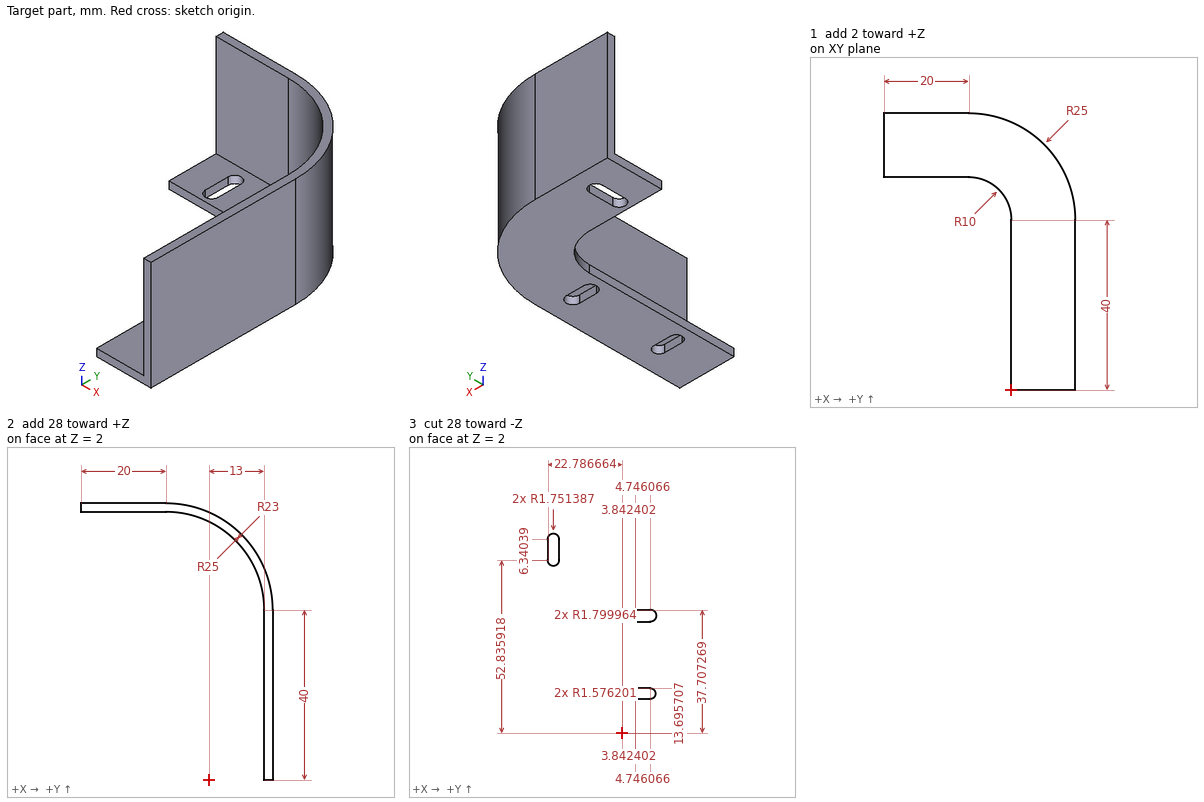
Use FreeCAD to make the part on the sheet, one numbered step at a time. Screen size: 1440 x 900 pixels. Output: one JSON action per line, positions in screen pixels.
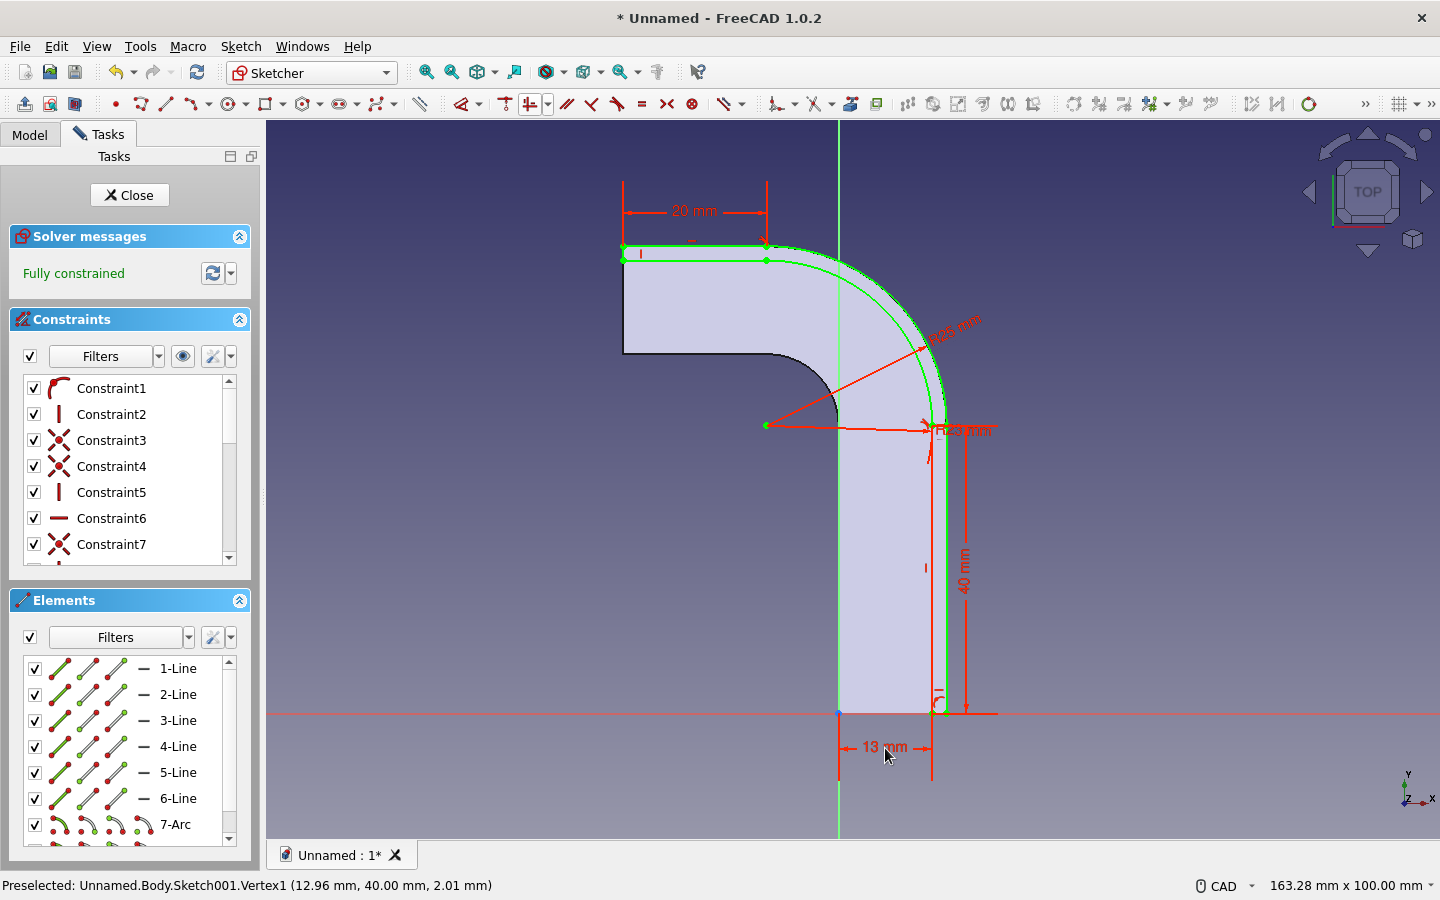
{"action": "left_click", "coordinate": [130, 195]}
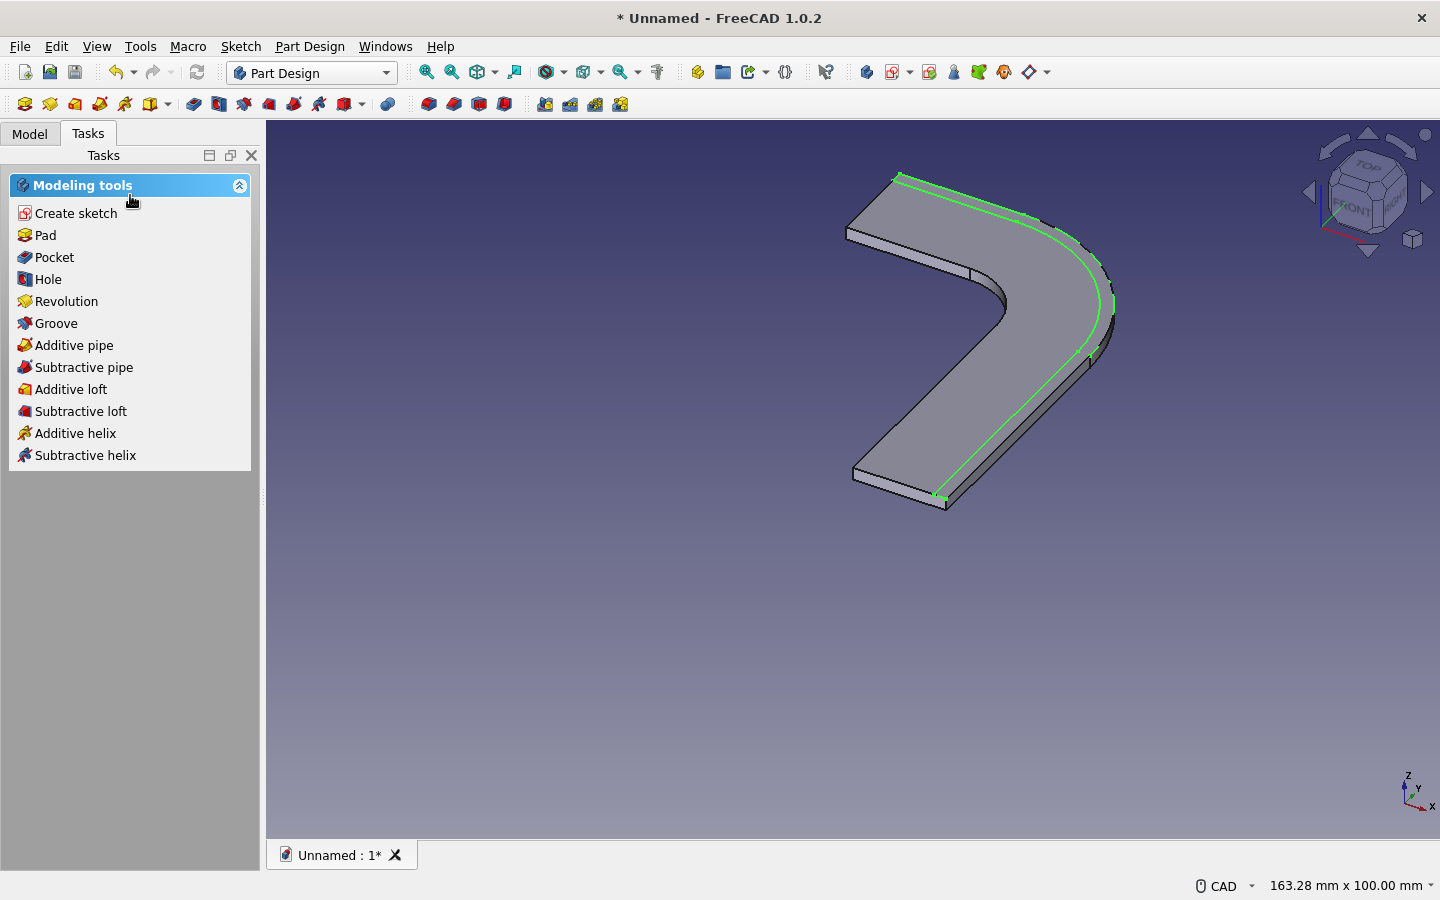
{"action": "left_click", "coordinate": [25, 104]}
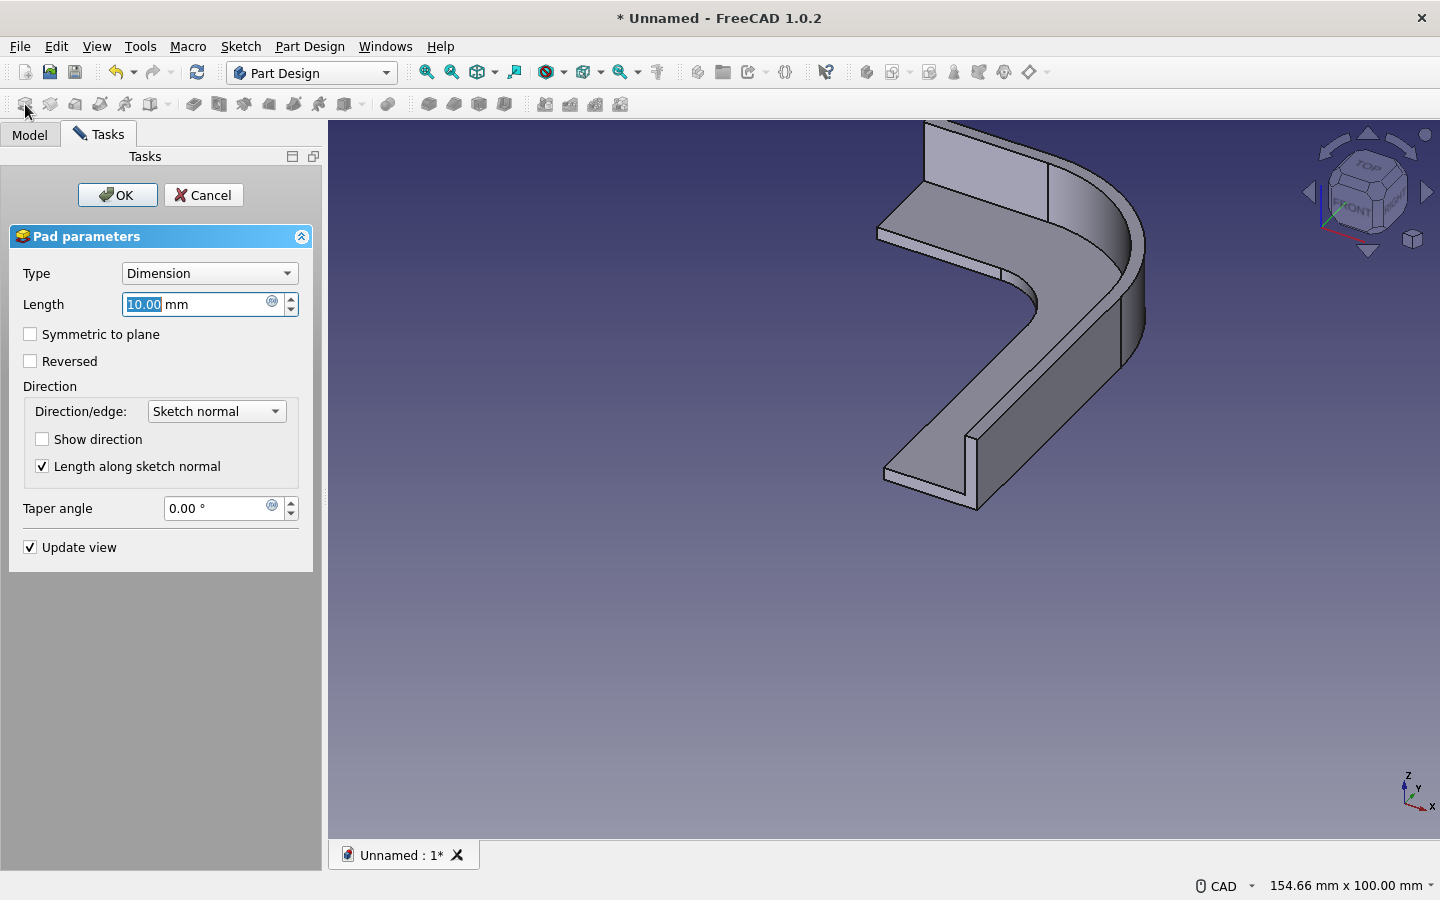
{"action": "type", "text": "28"}
{"action": "key", "text": "Tab"}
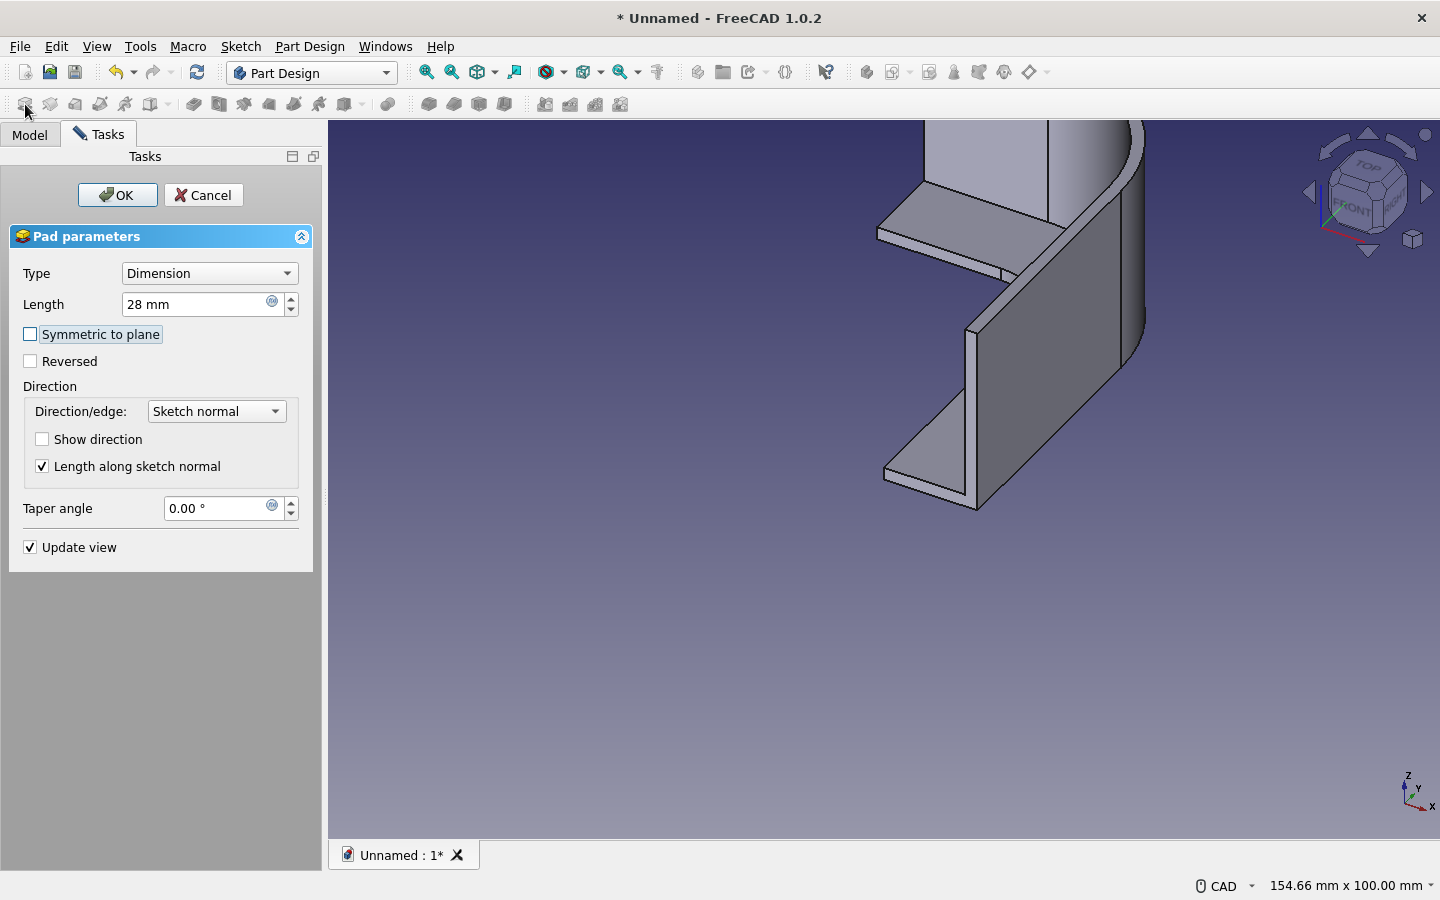
{"action": "left_click", "coordinate": [118, 195]}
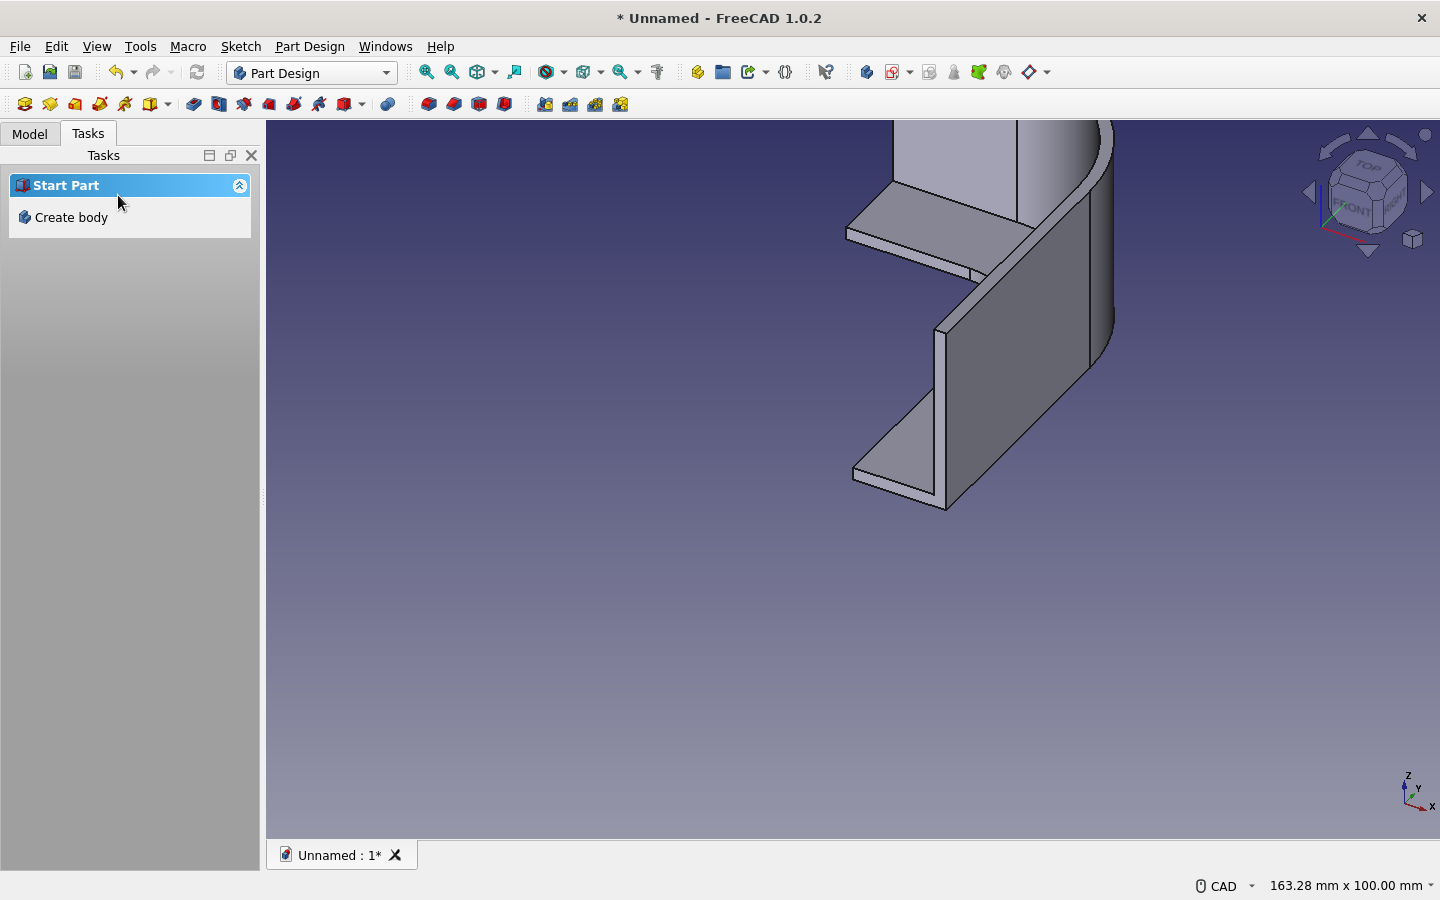
{"action": "left_click", "coordinate": [427, 72]}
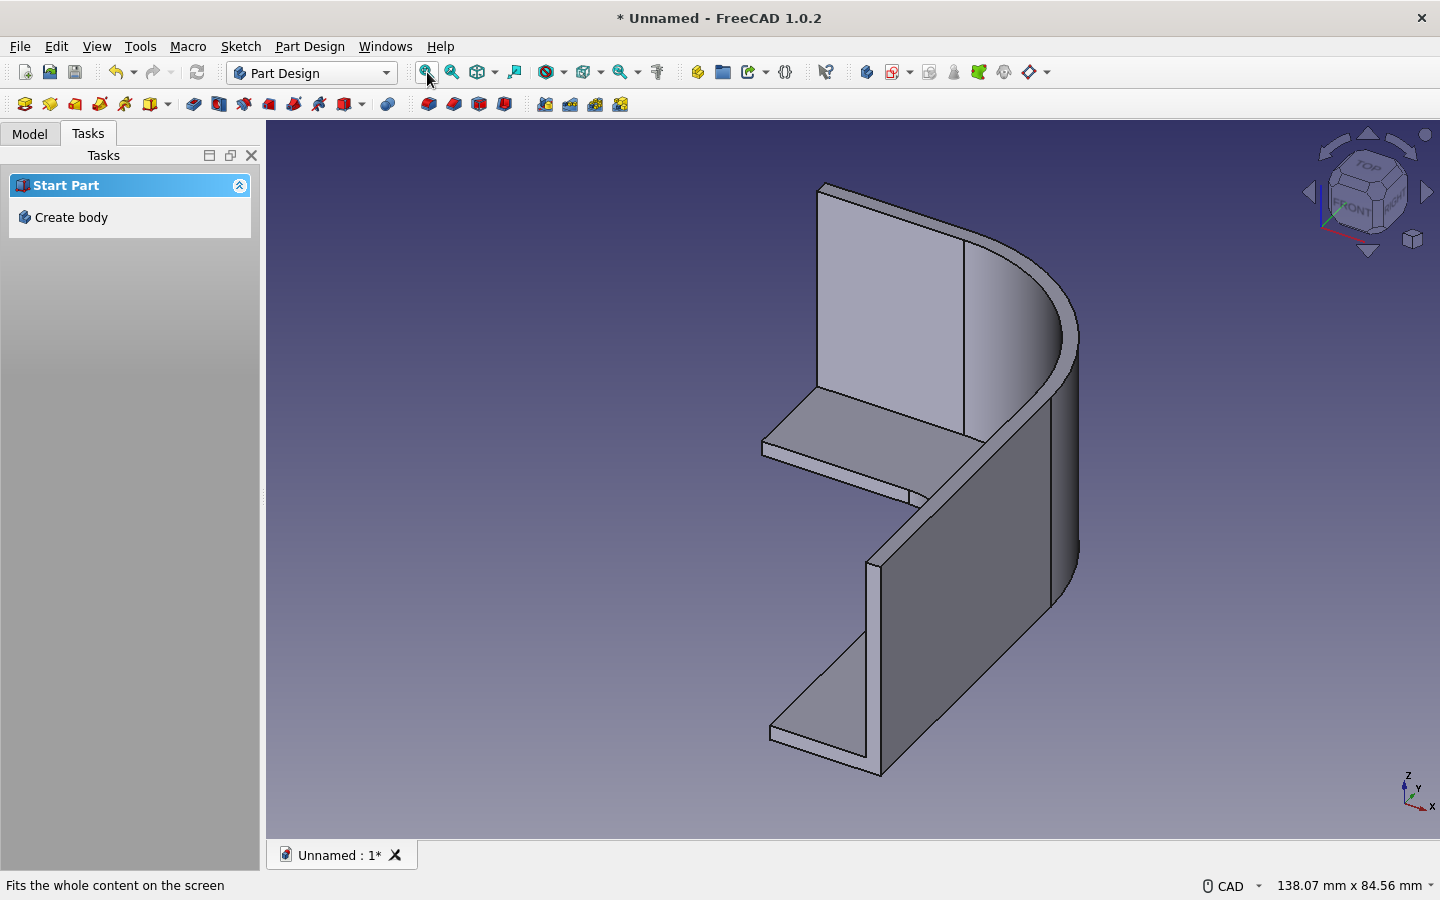
{"action": "left_click", "coordinate": [911, 442]}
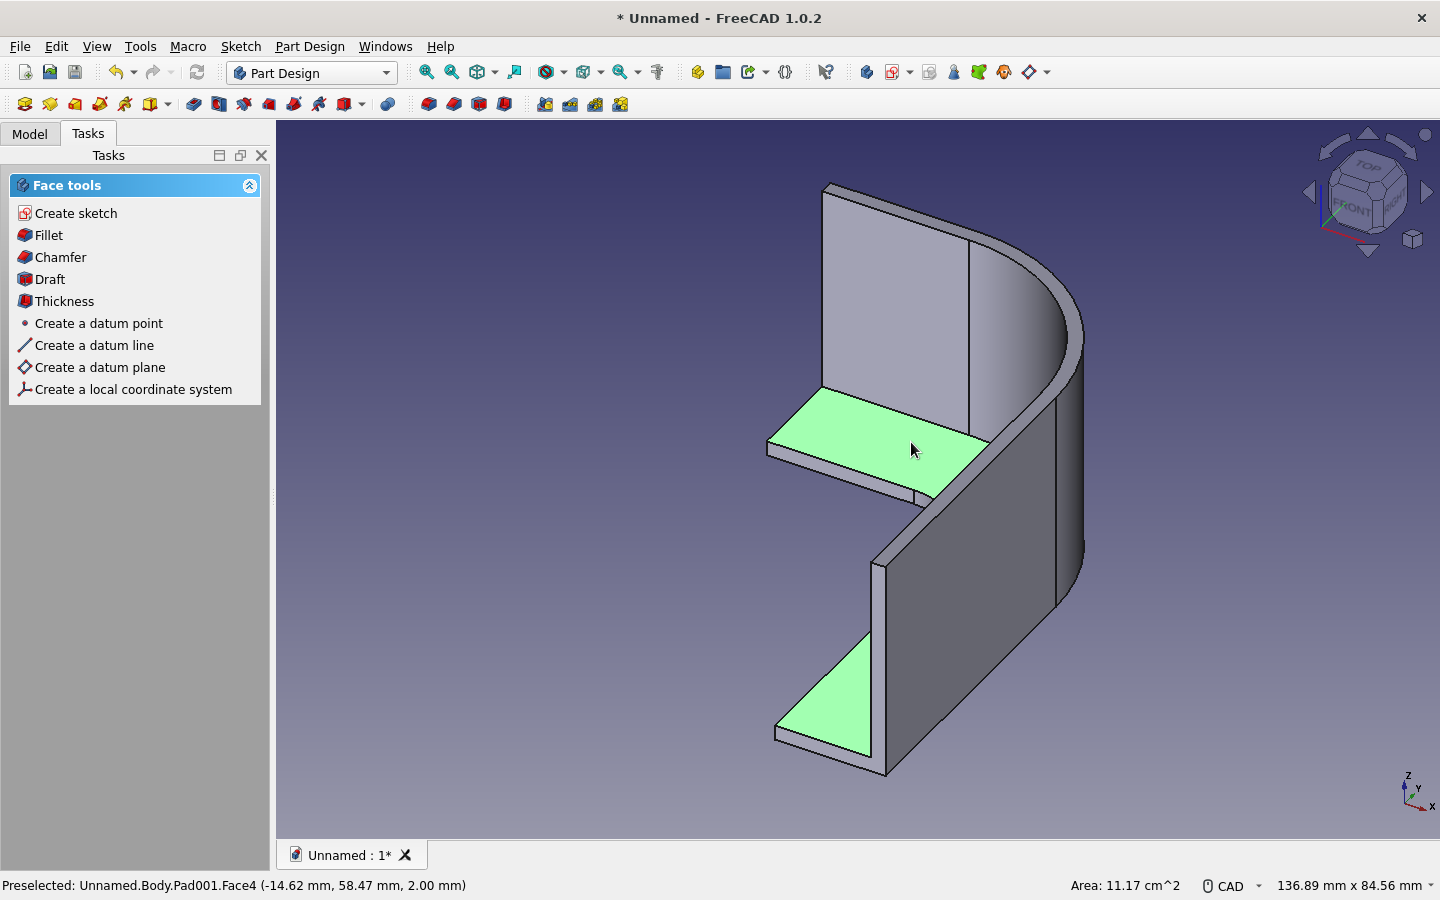
{"action": "left_click", "coordinate": [892, 72]}